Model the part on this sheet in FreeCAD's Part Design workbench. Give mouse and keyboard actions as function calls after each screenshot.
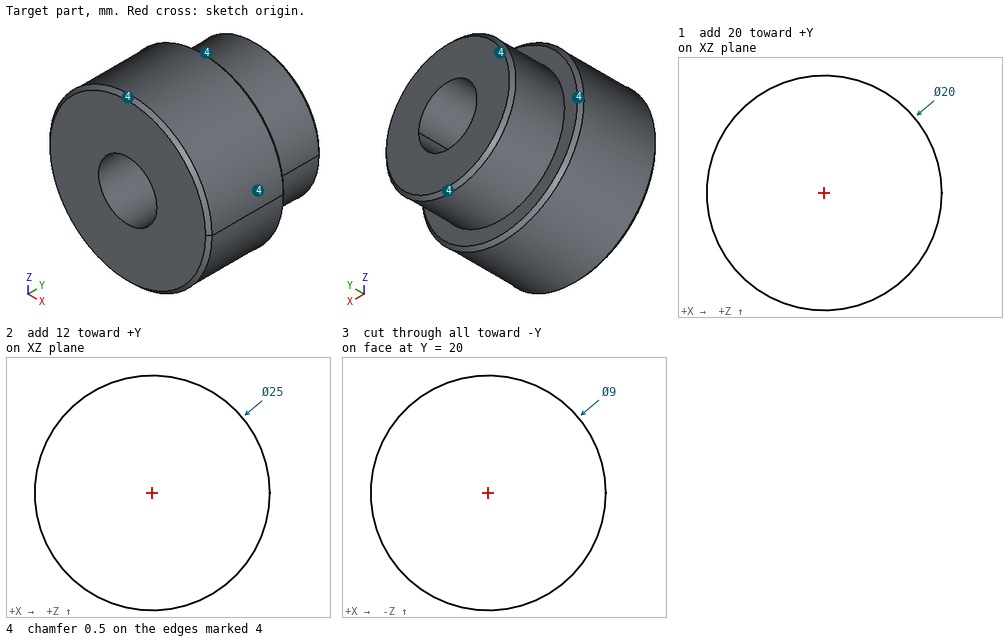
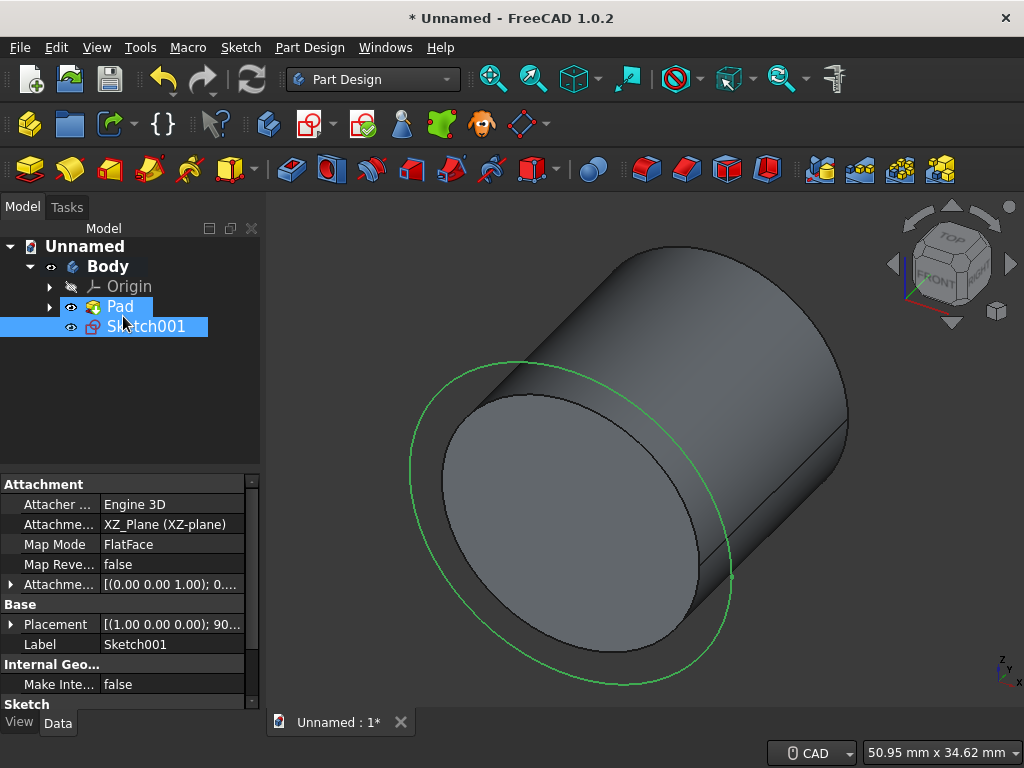
click(30, 170)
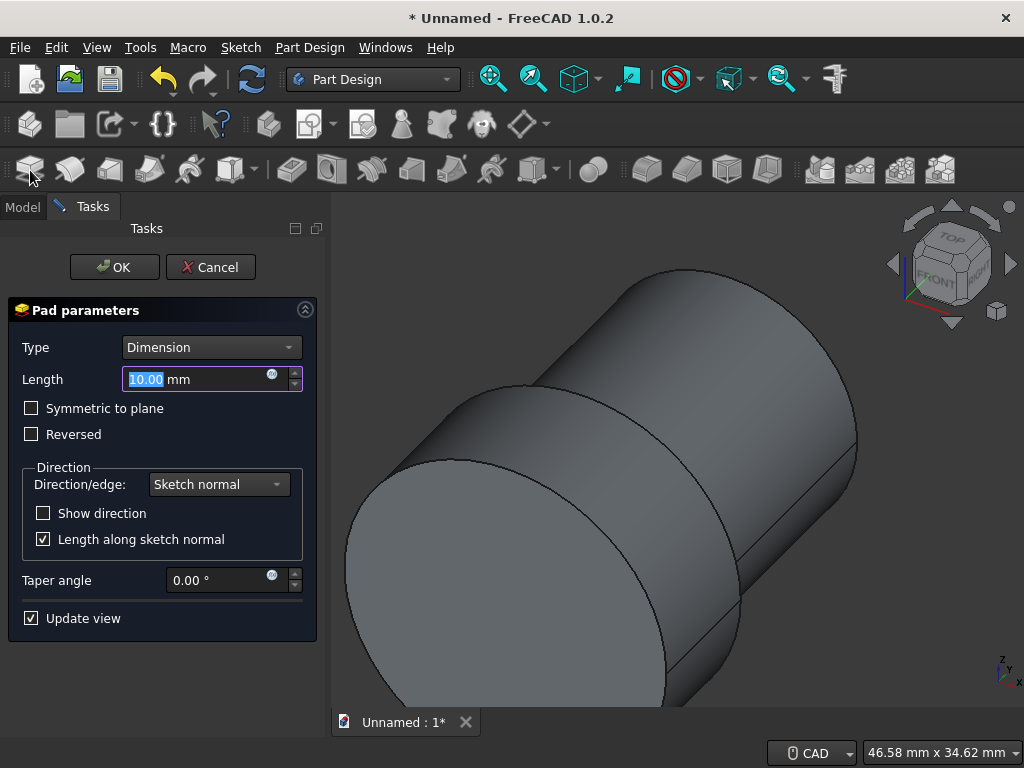
text(12)
key(Tab)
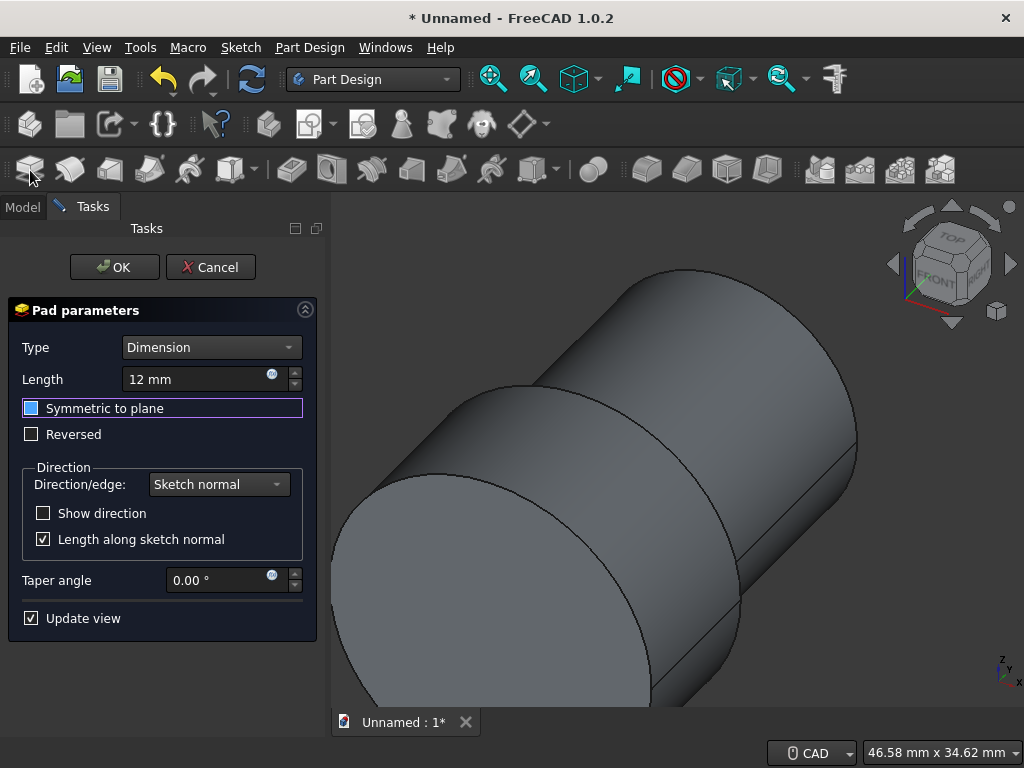
click(30, 434)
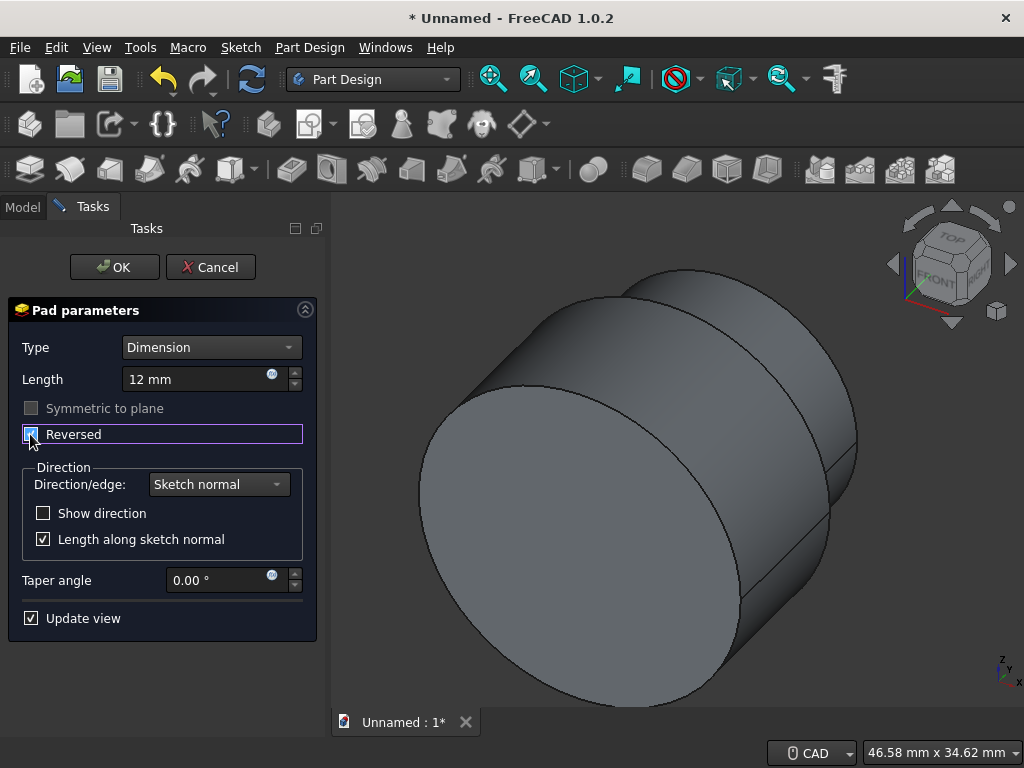
click(115, 267)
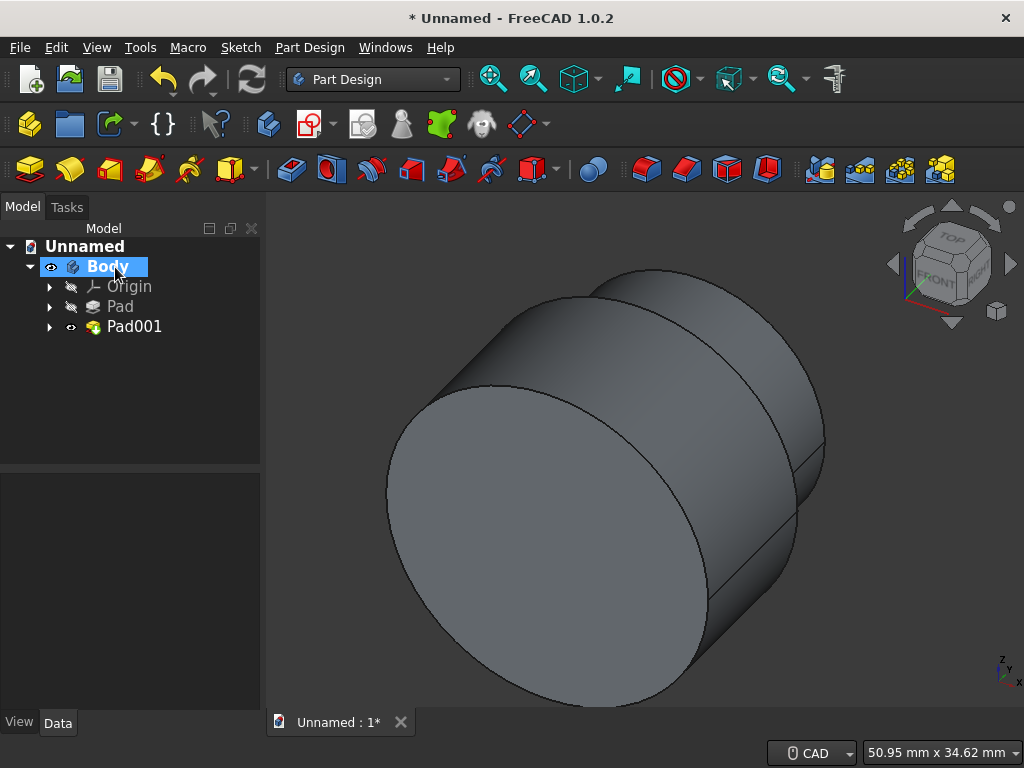
click(494, 80)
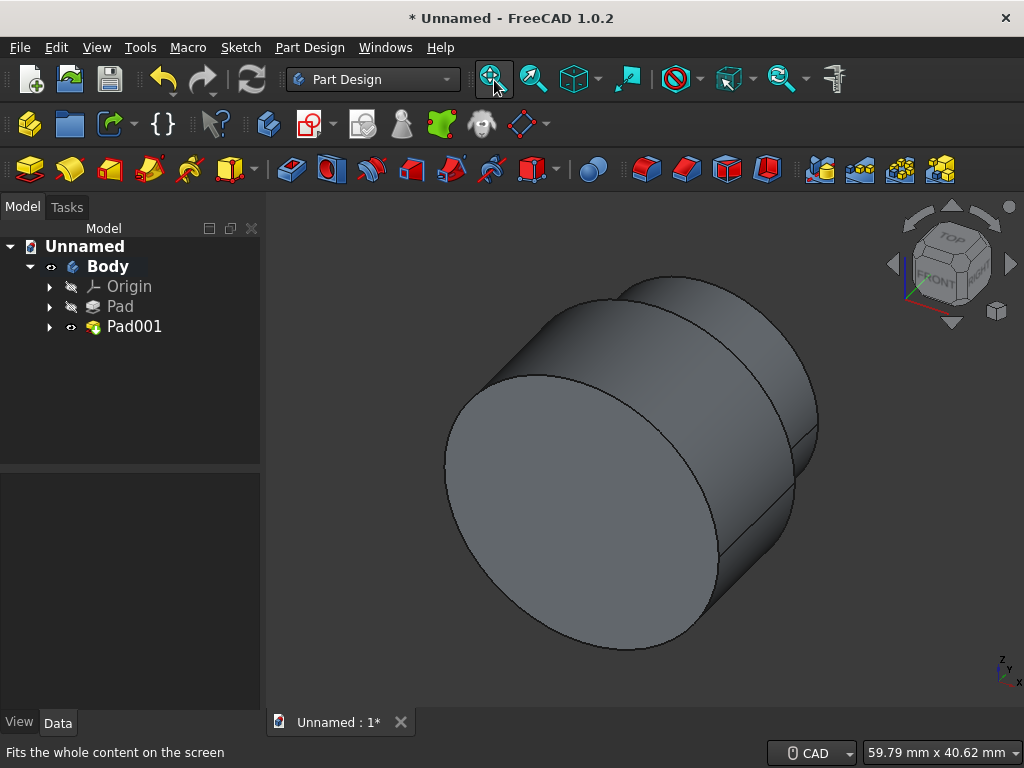
key(4)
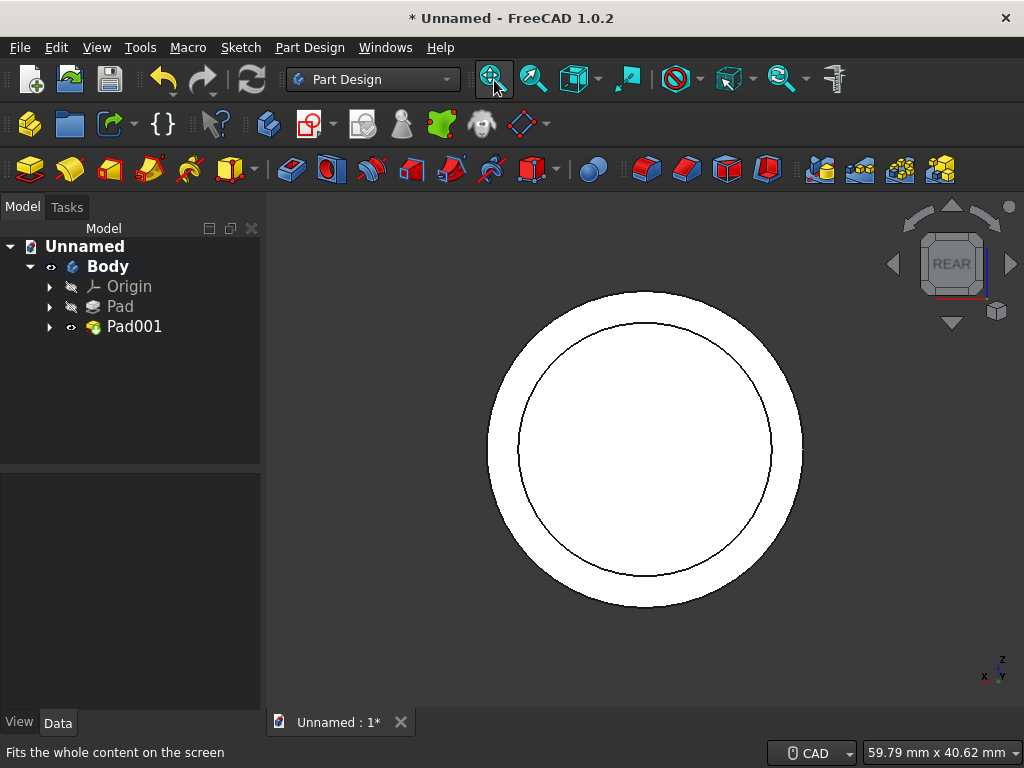
click(645, 449)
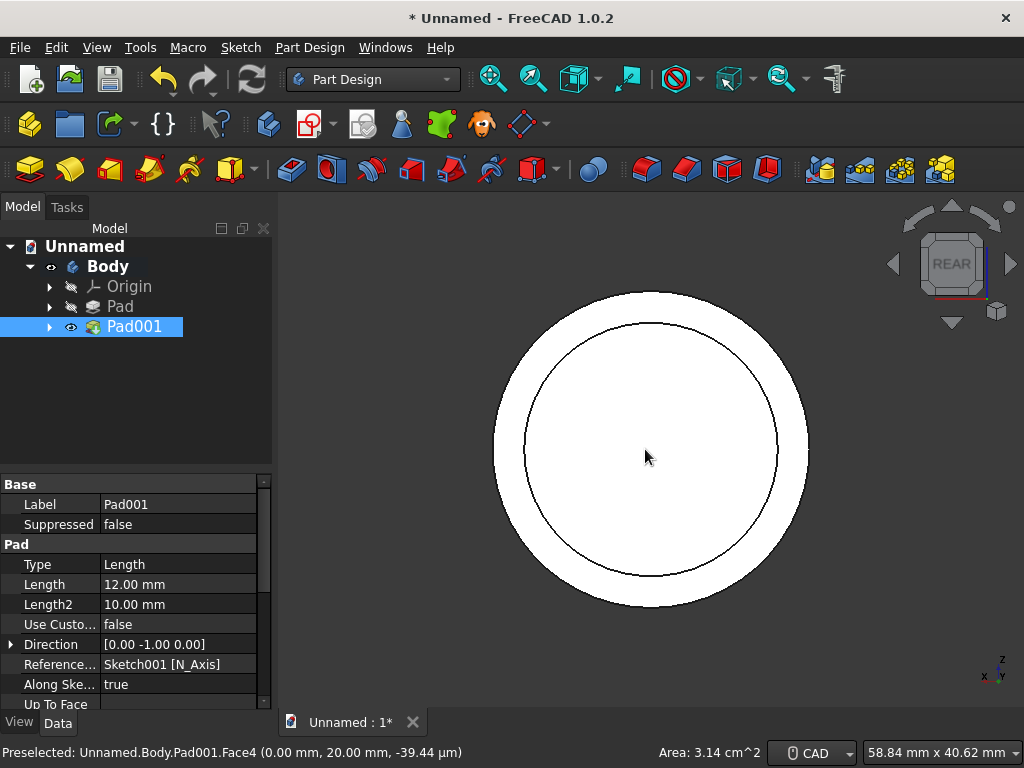
click(310, 124)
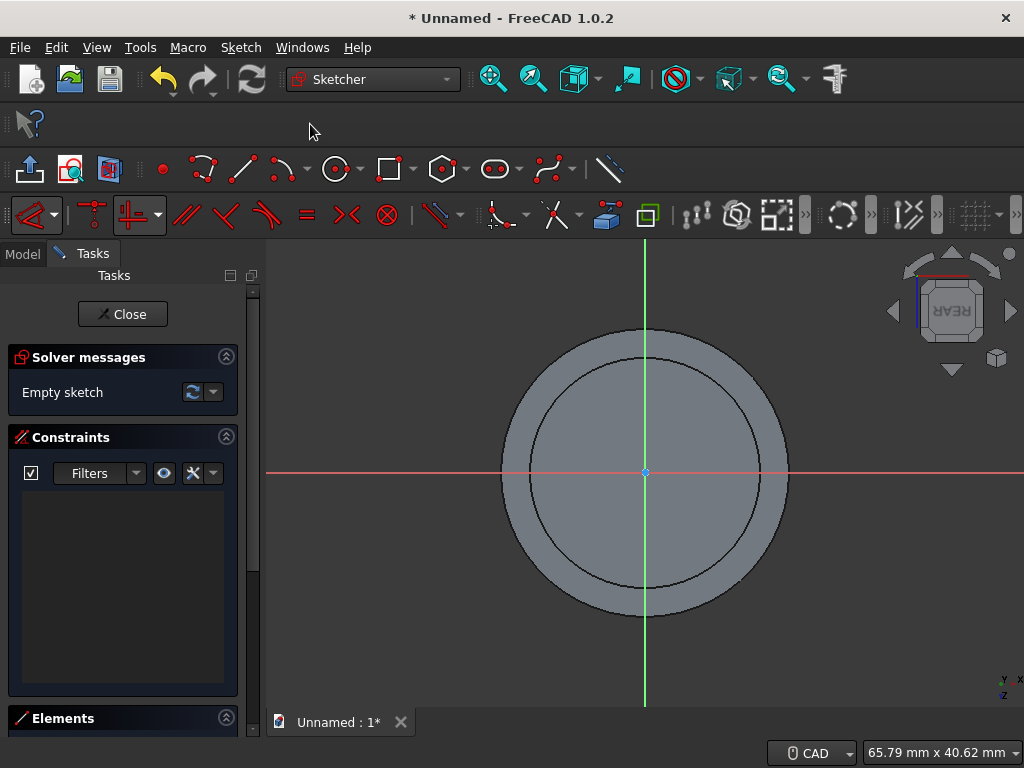
scroll(685, 473, up, 5)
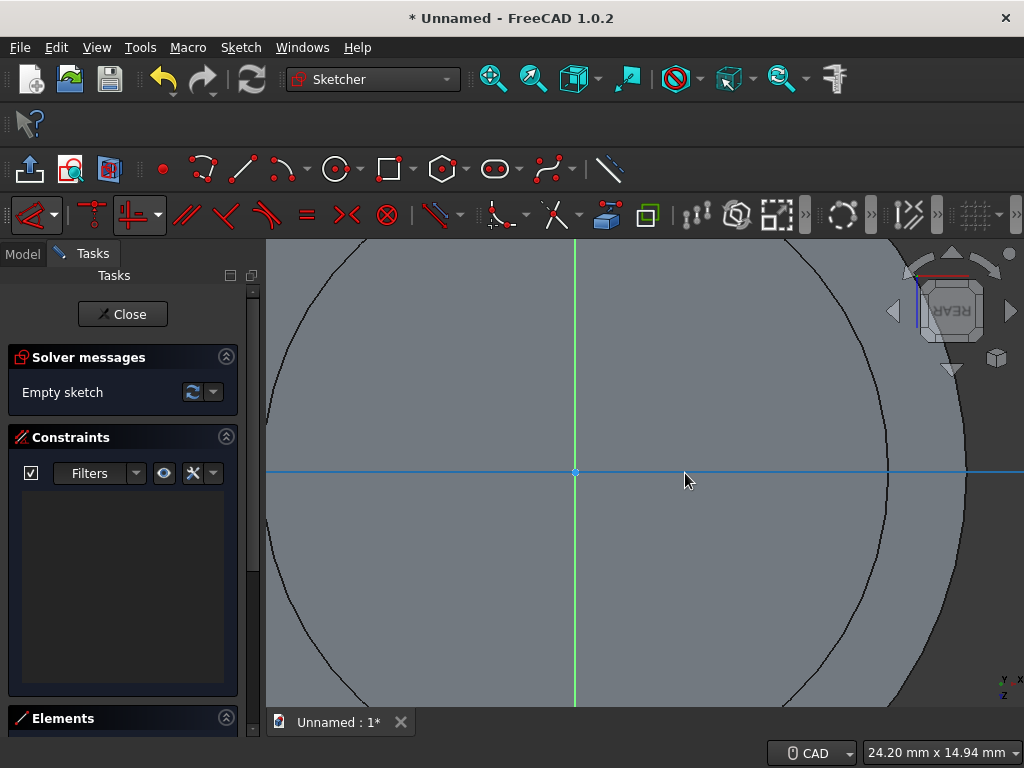
click(336, 170)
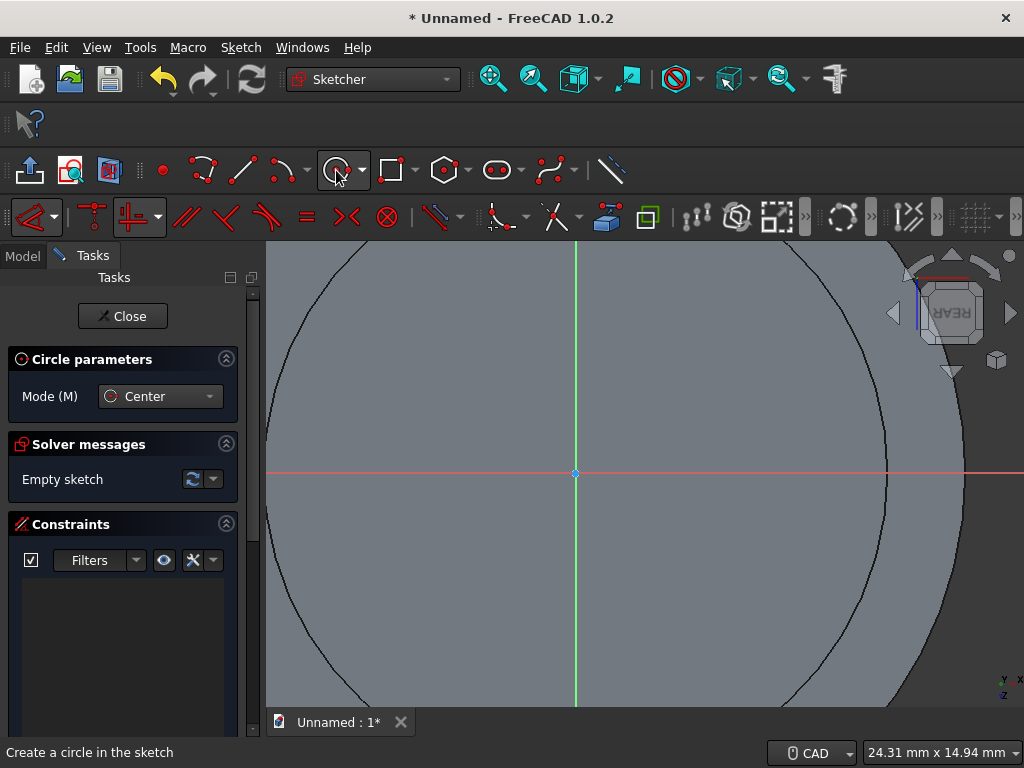
click(576, 473)
click(675, 374)
key(Escape)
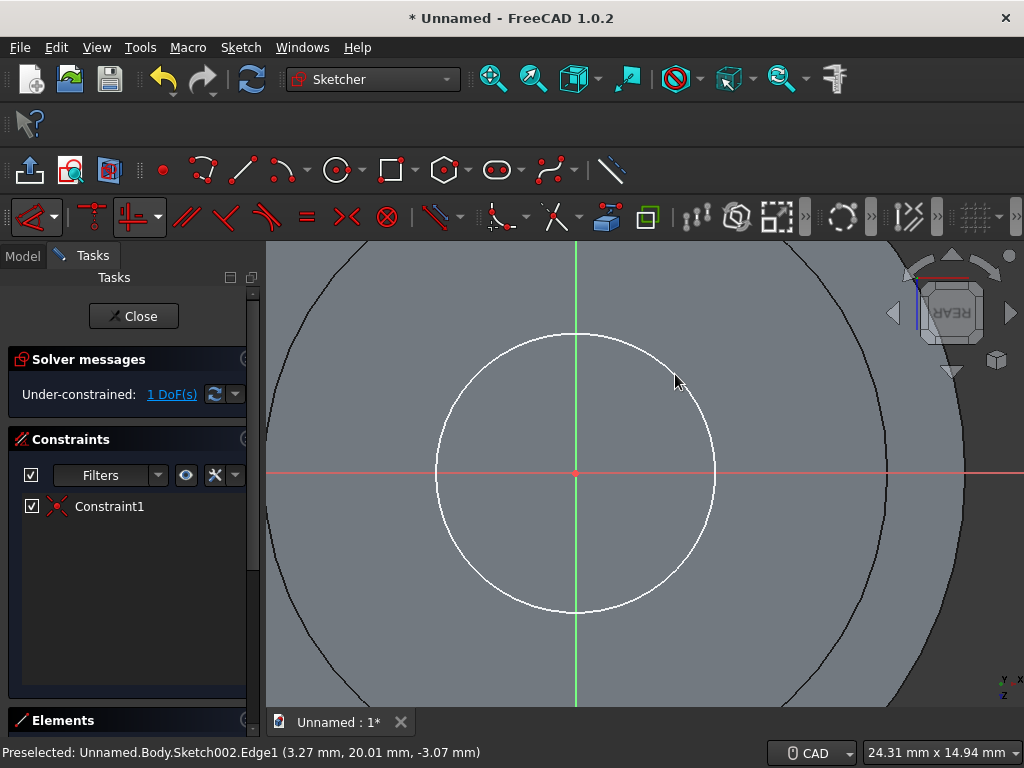
click(674, 374)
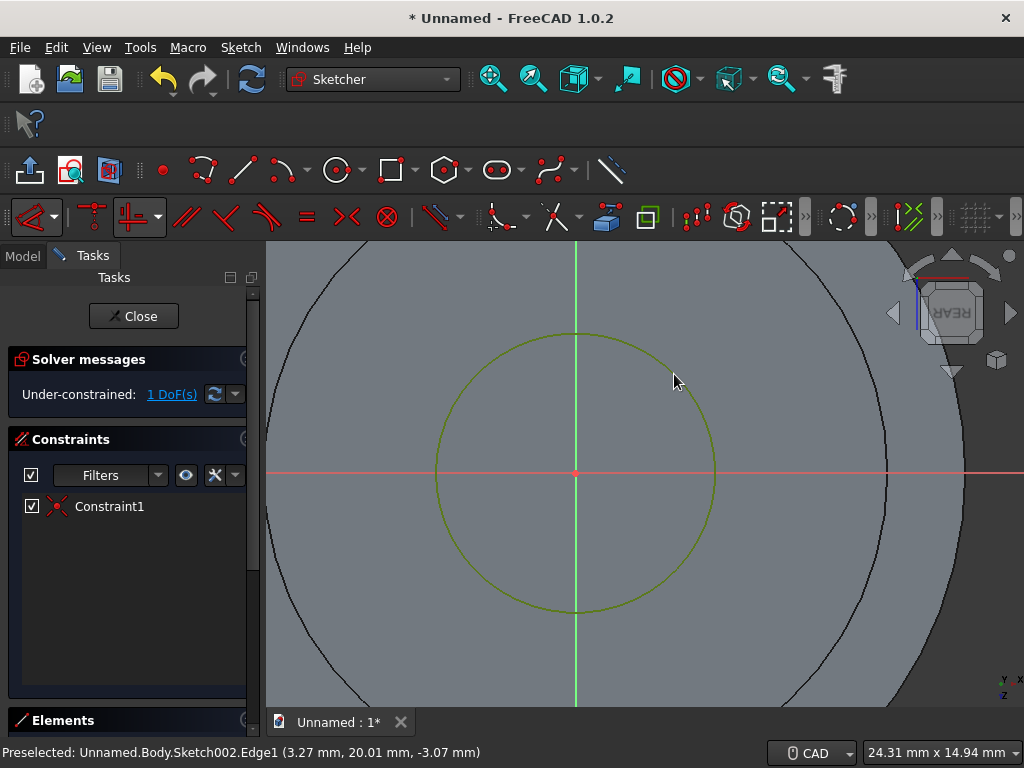
click(56, 218)